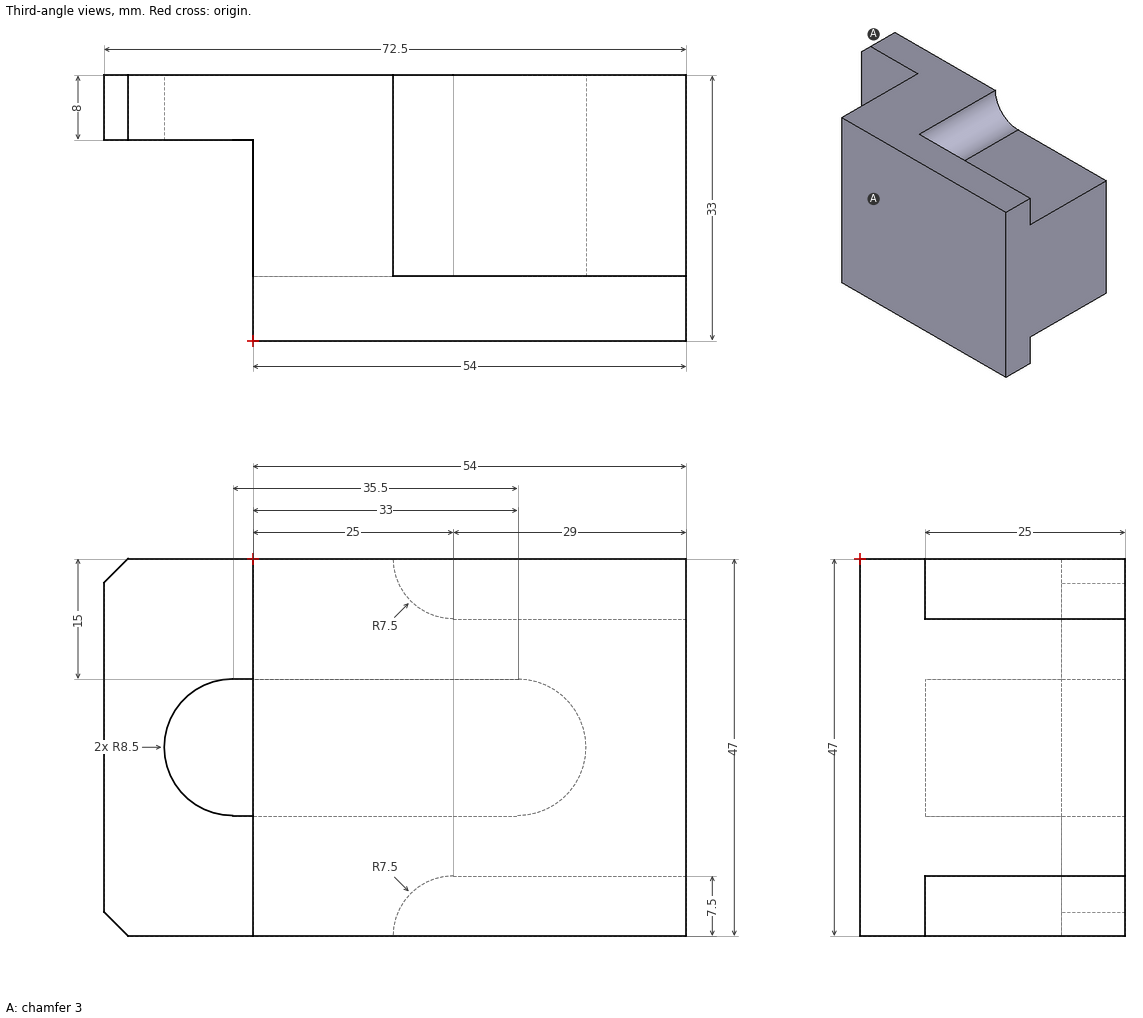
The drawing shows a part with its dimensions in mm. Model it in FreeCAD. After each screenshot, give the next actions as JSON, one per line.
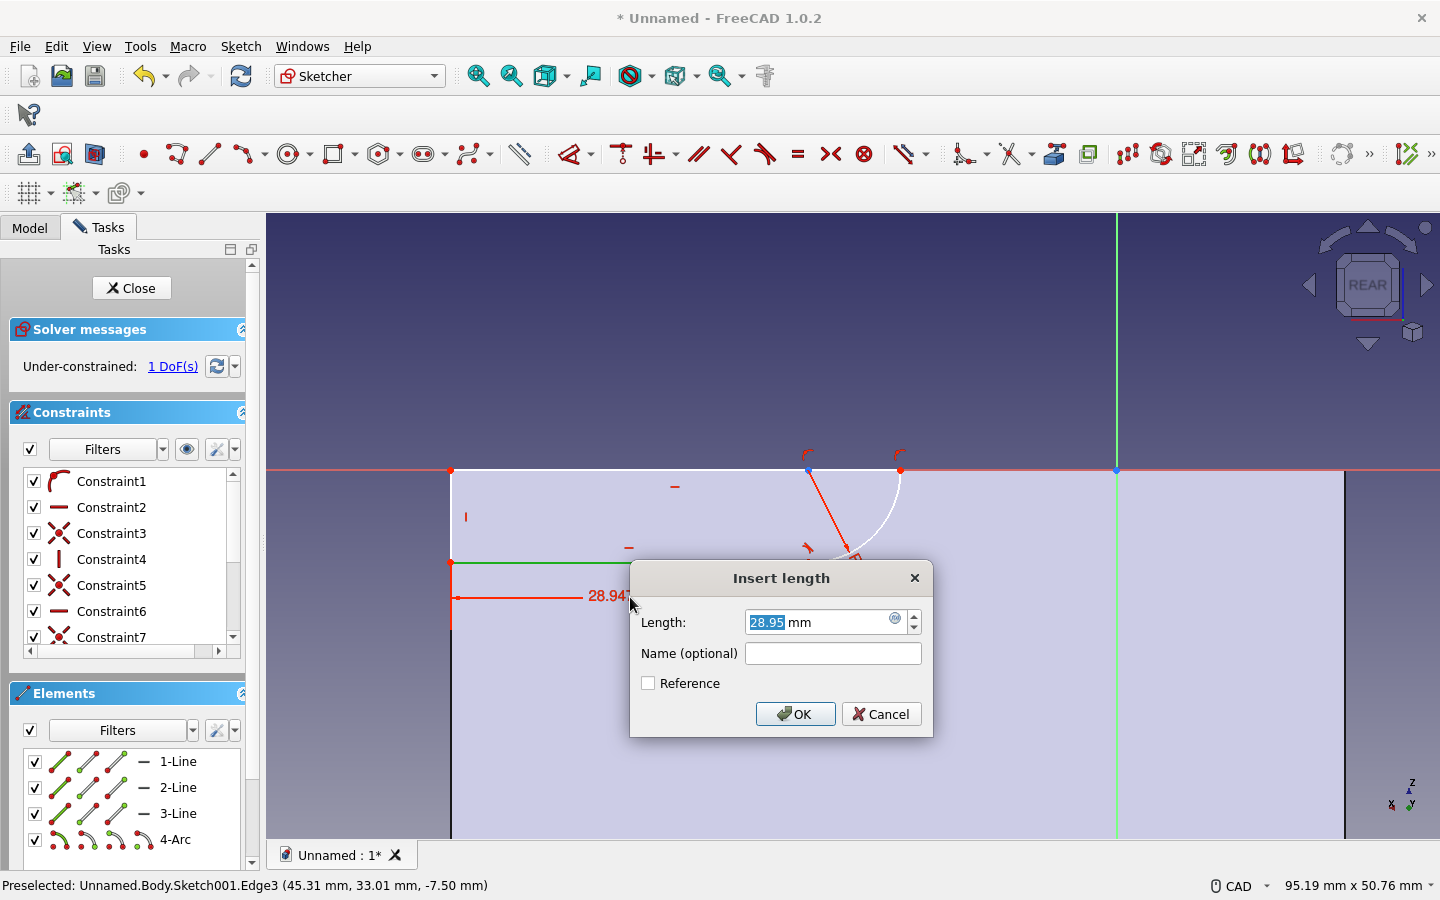
{"action": "type", "text": "29"}
{"action": "key", "text": "Return"}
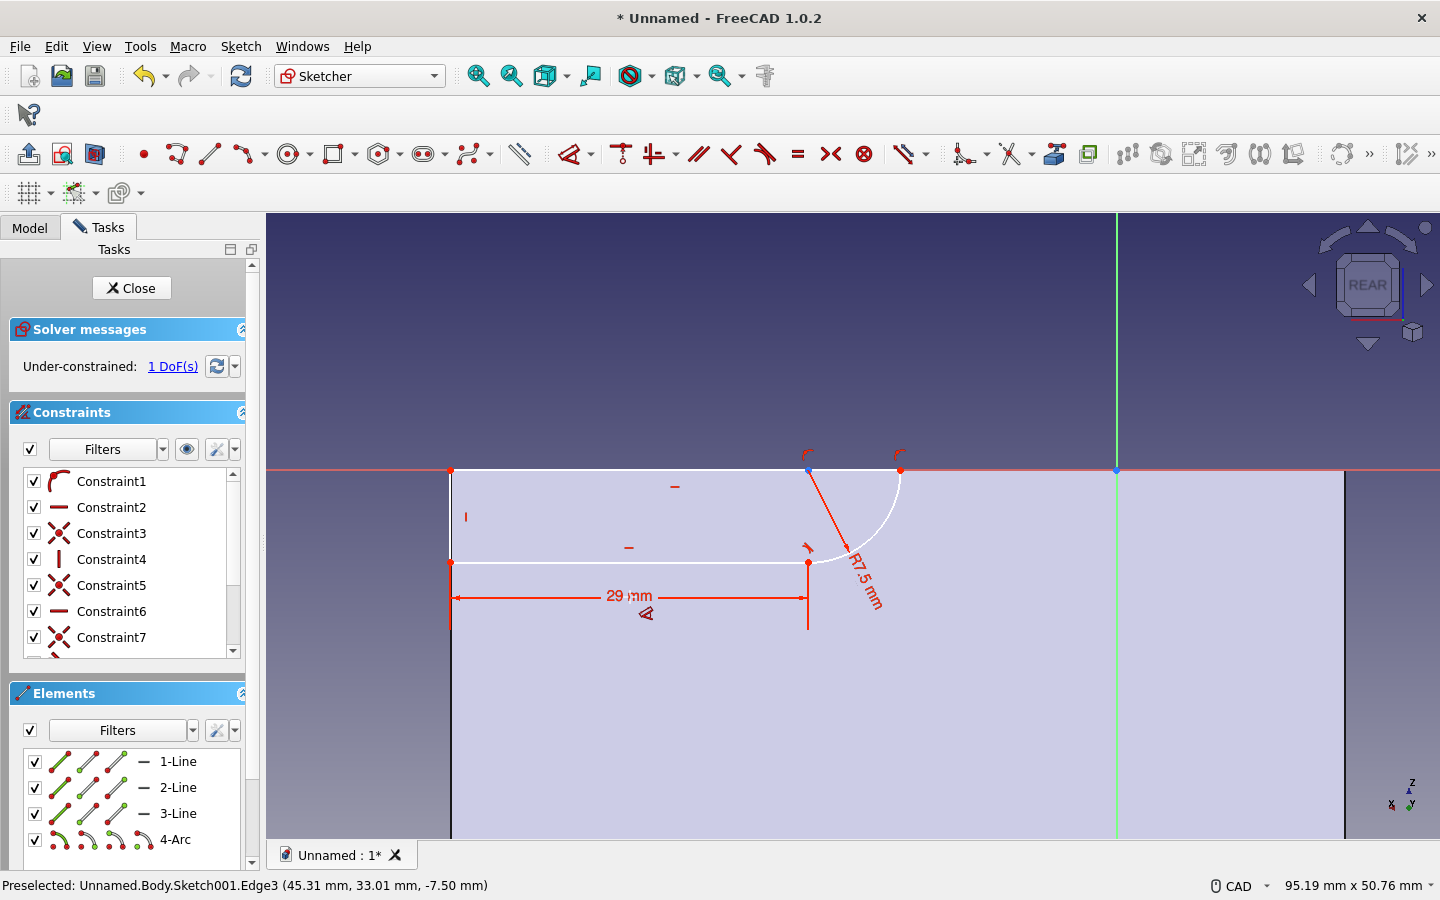
{"action": "left_click", "coordinate": [450, 470]}
{"action": "left_click", "coordinate": [784, 436]}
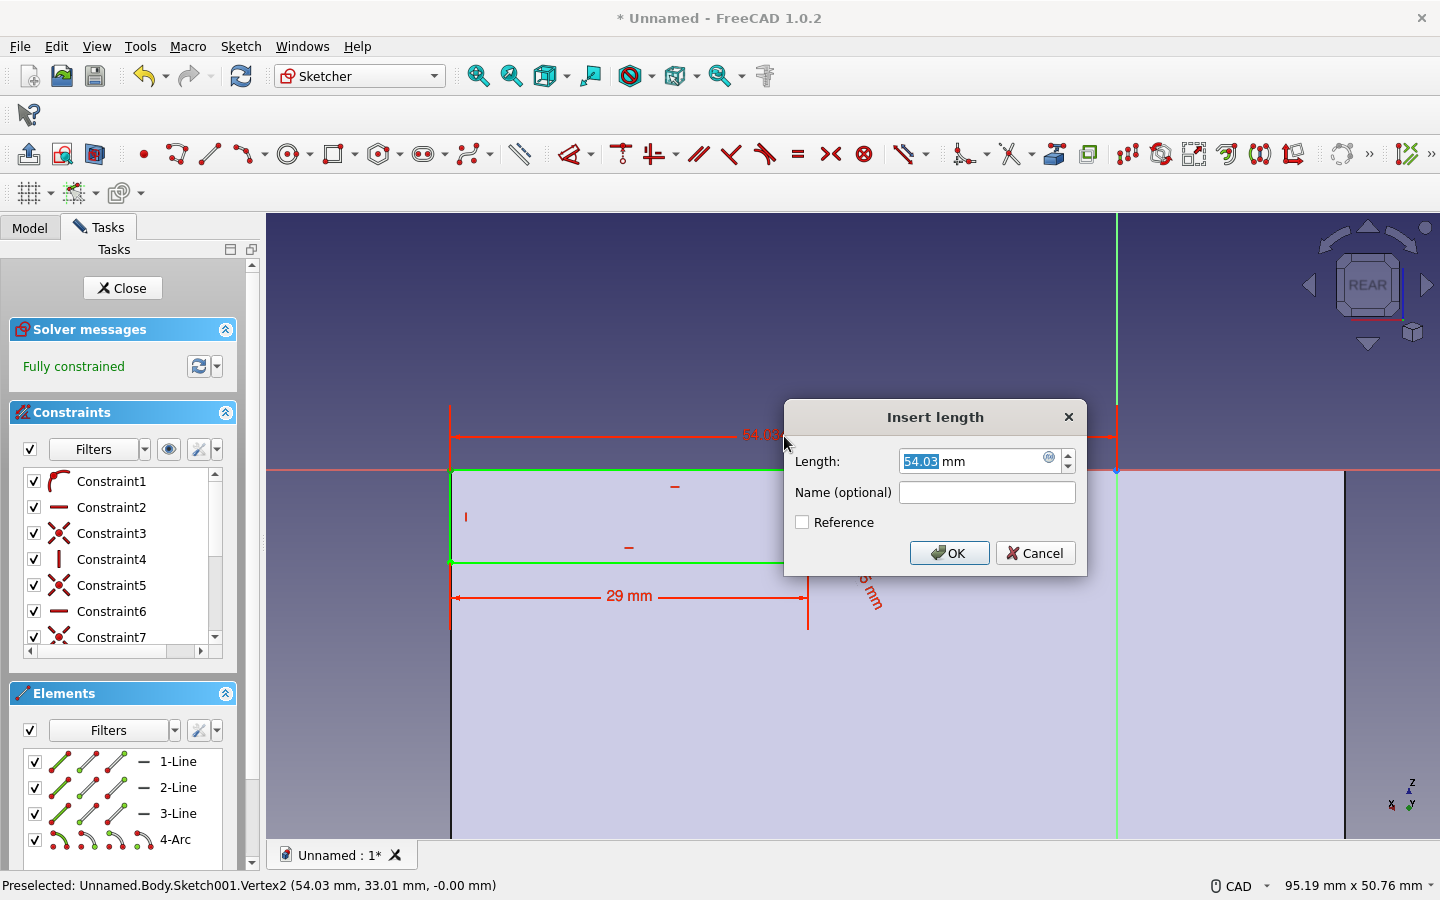
{"action": "type", "text": "54"}
{"action": "key", "text": "Return"}
{"action": "key", "text": "Escape"}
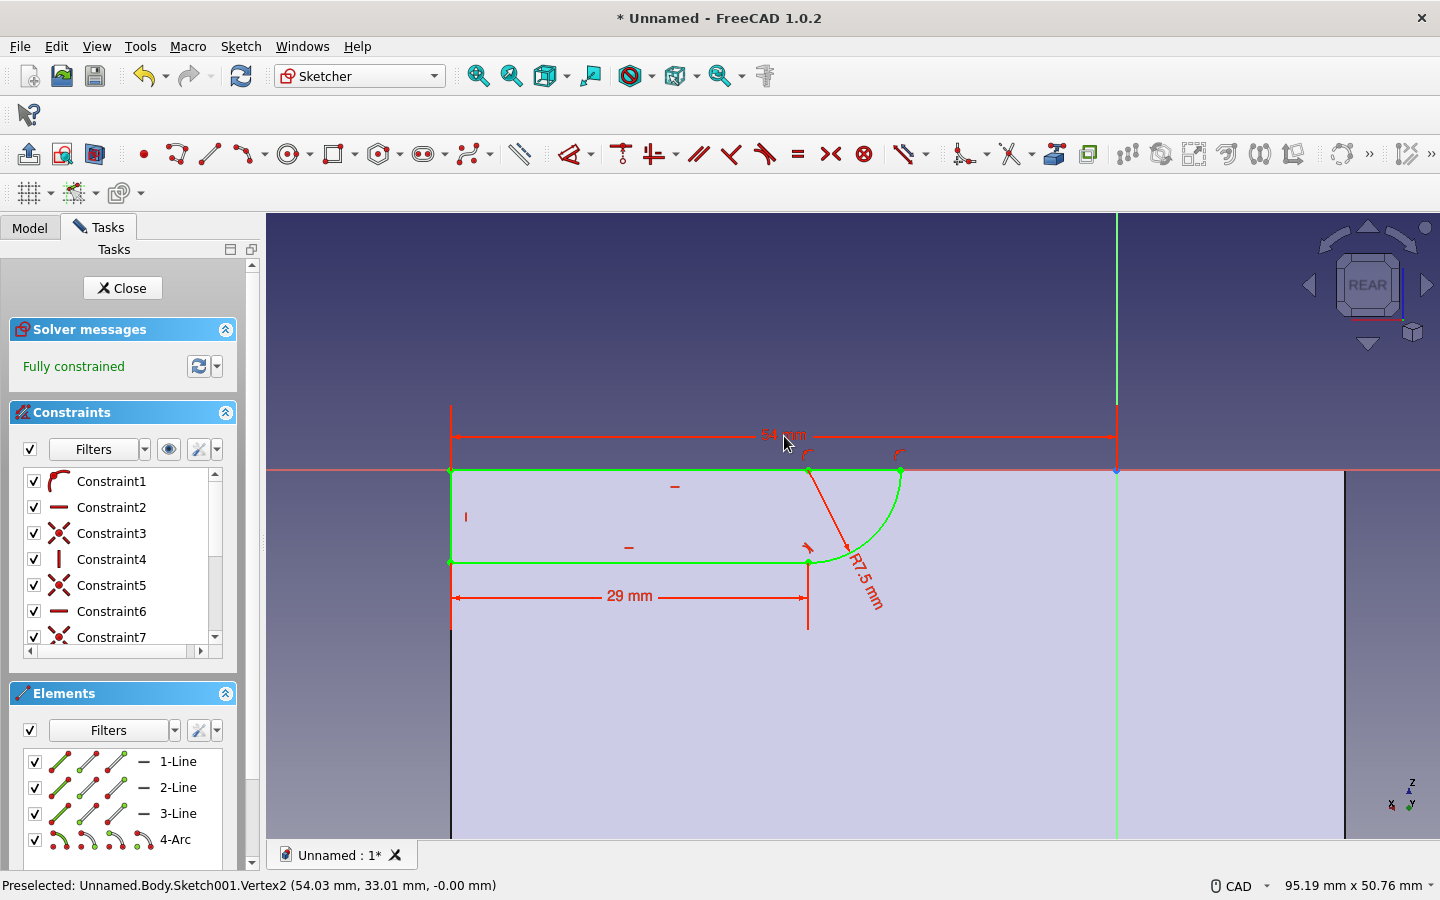
{"action": "left_click", "coordinate": [123, 288]}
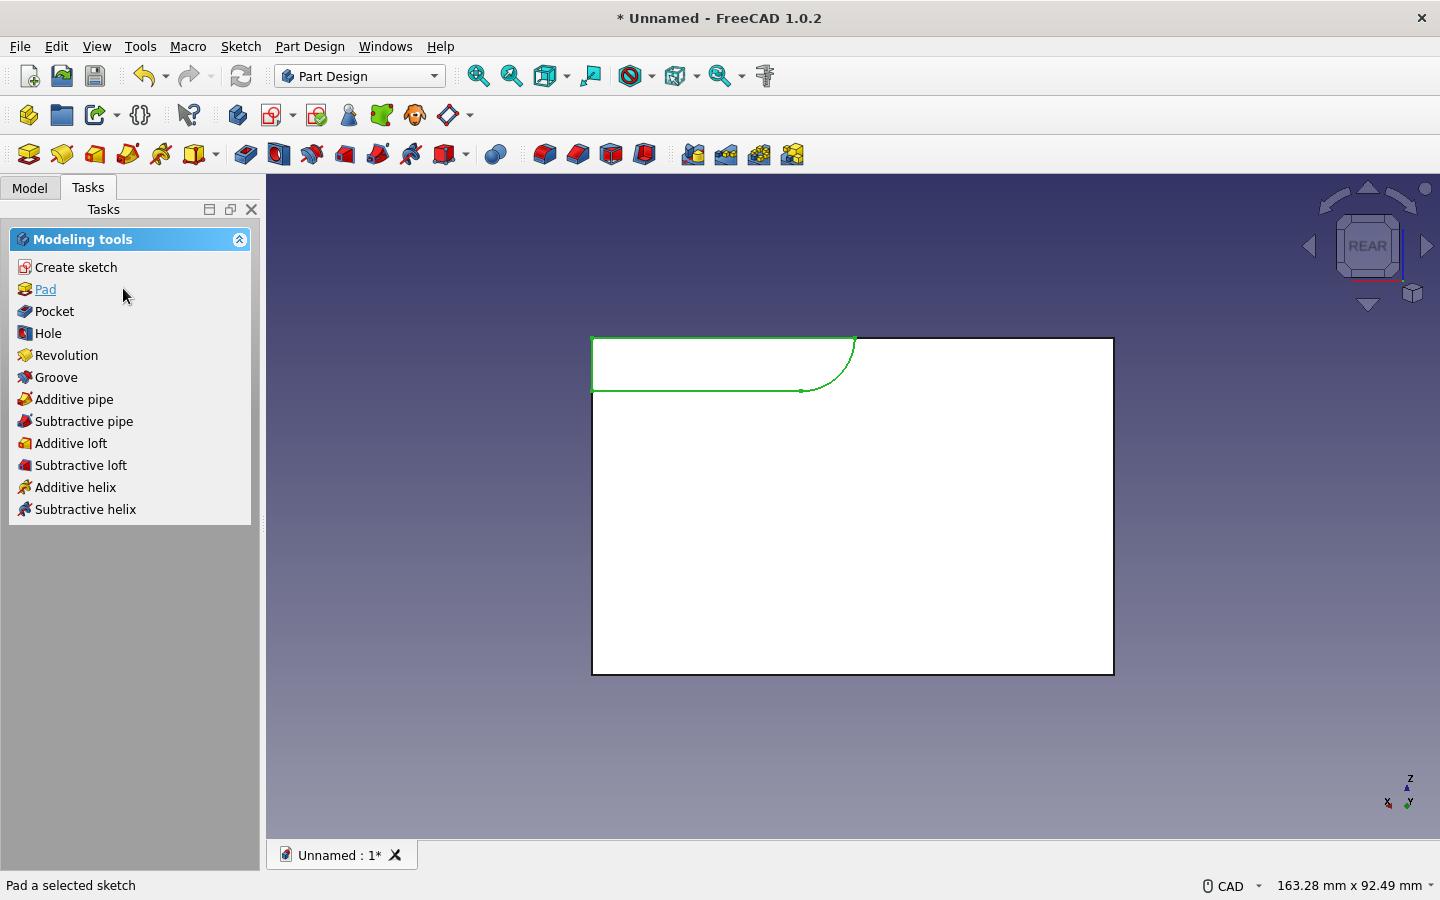
{"action": "left_click", "coordinate": [246, 154]}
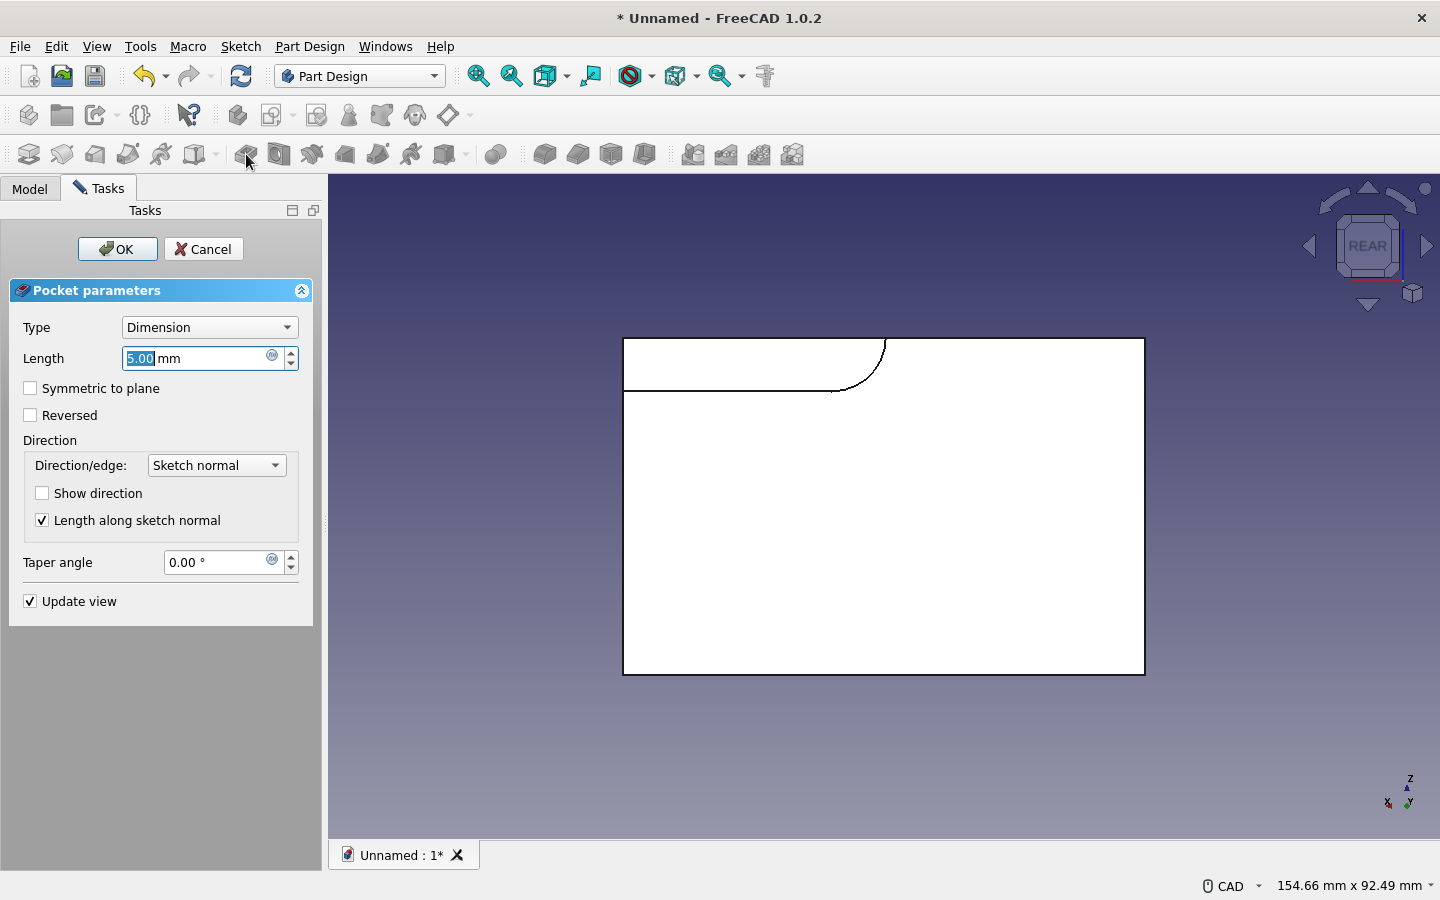
{"action": "type", "text": "25"}
{"action": "key", "text": "Tab"}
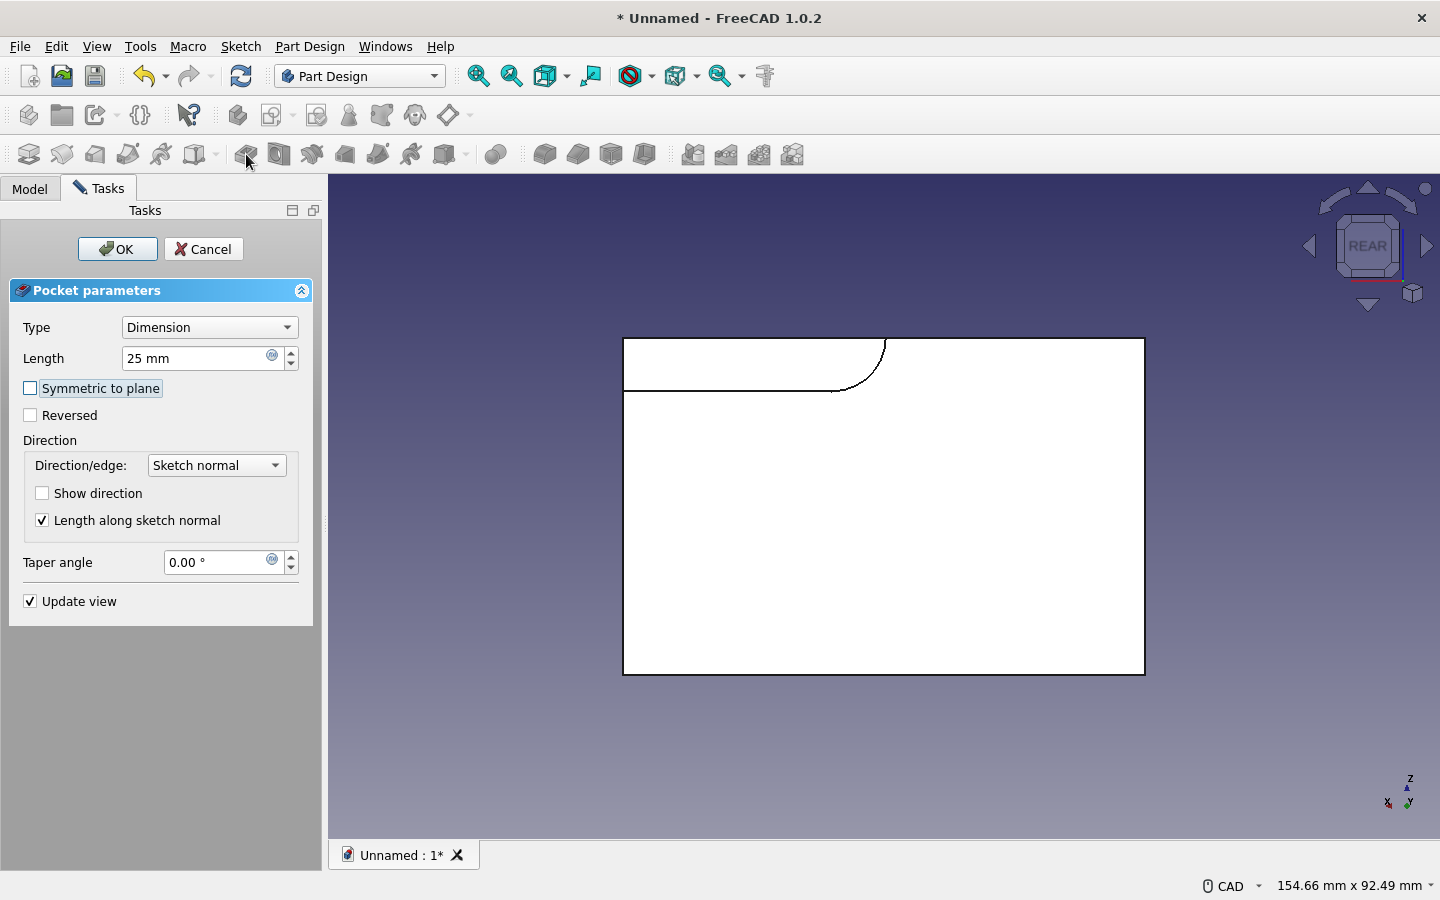
{"action": "left_click", "coordinate": [118, 249]}